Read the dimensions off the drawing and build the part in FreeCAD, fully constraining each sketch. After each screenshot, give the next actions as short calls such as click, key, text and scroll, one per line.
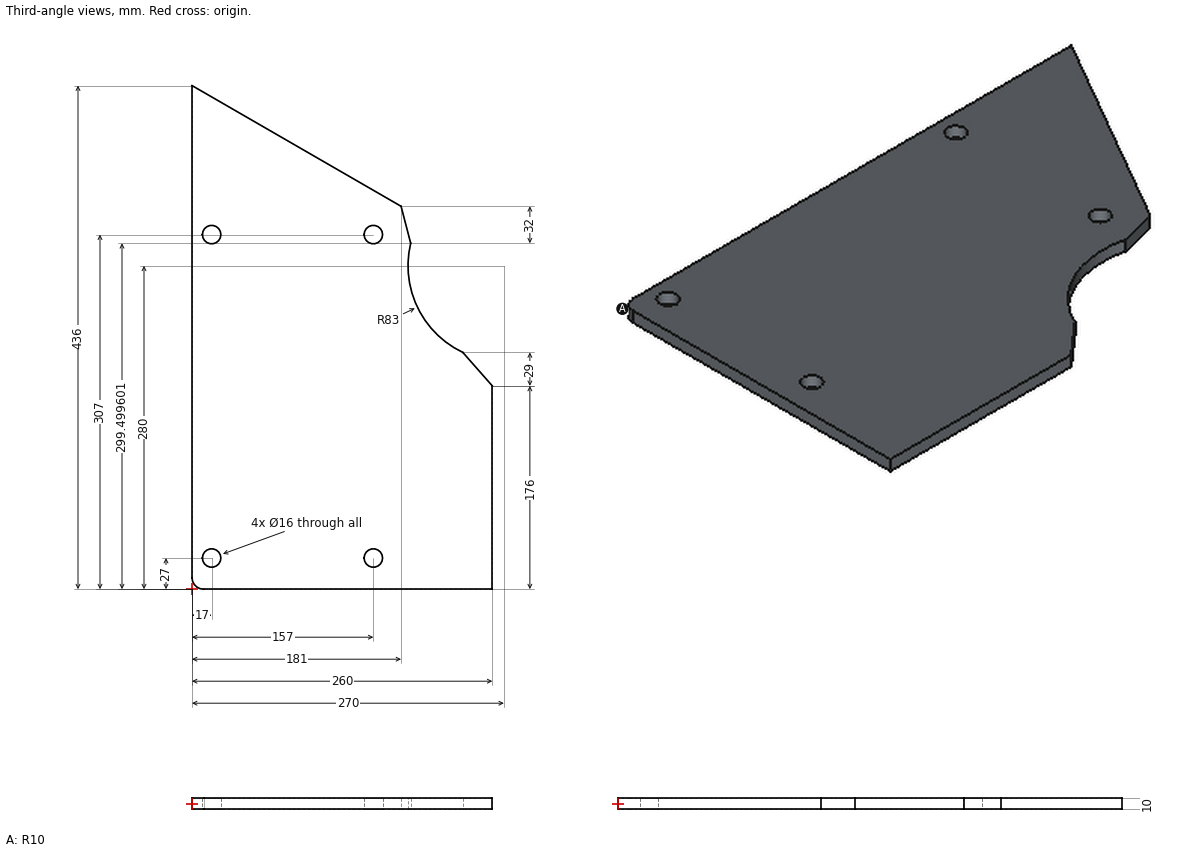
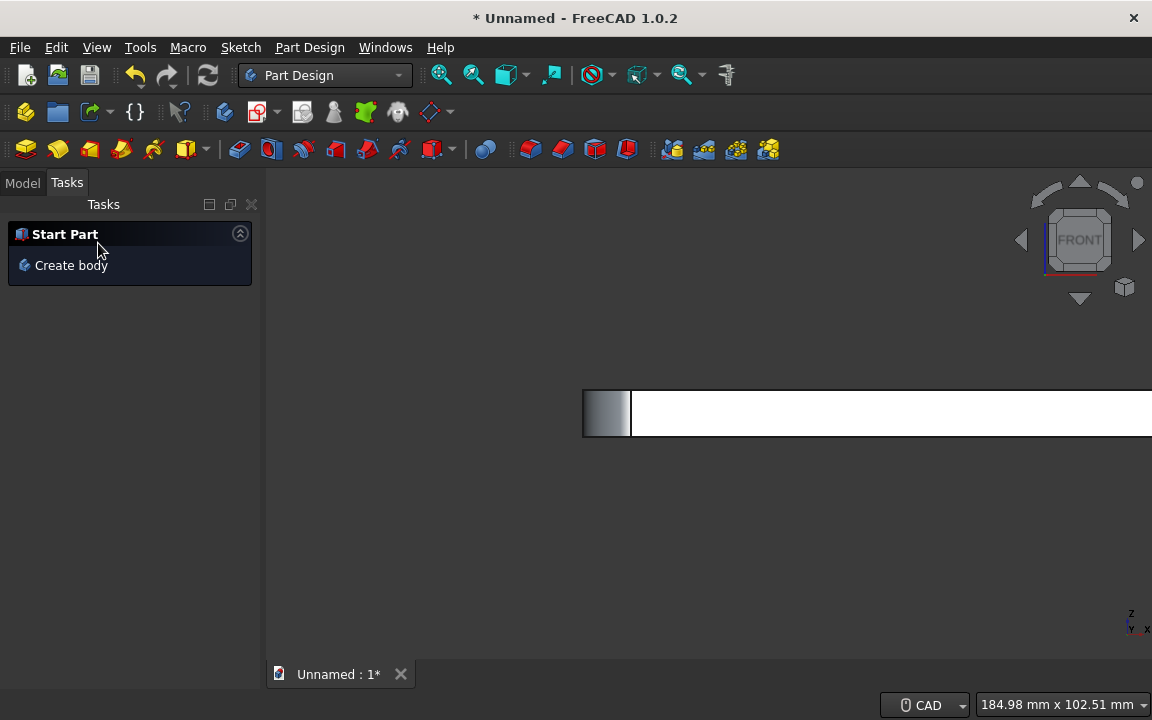
key(0)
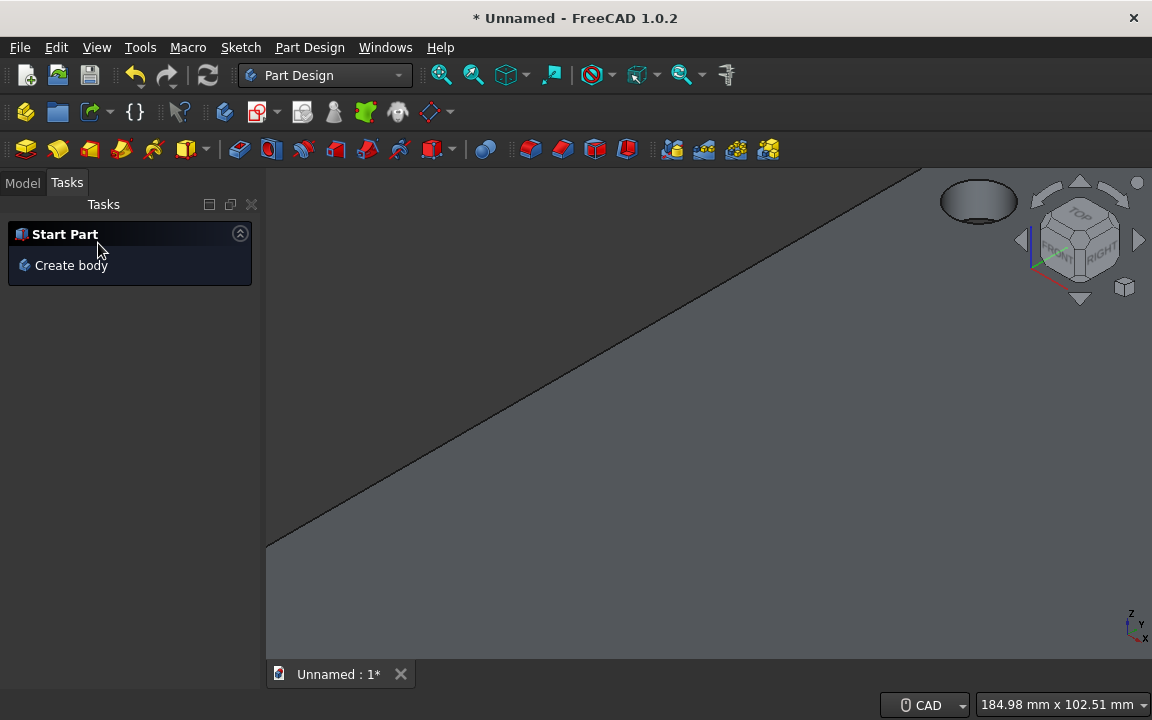
click(442, 76)